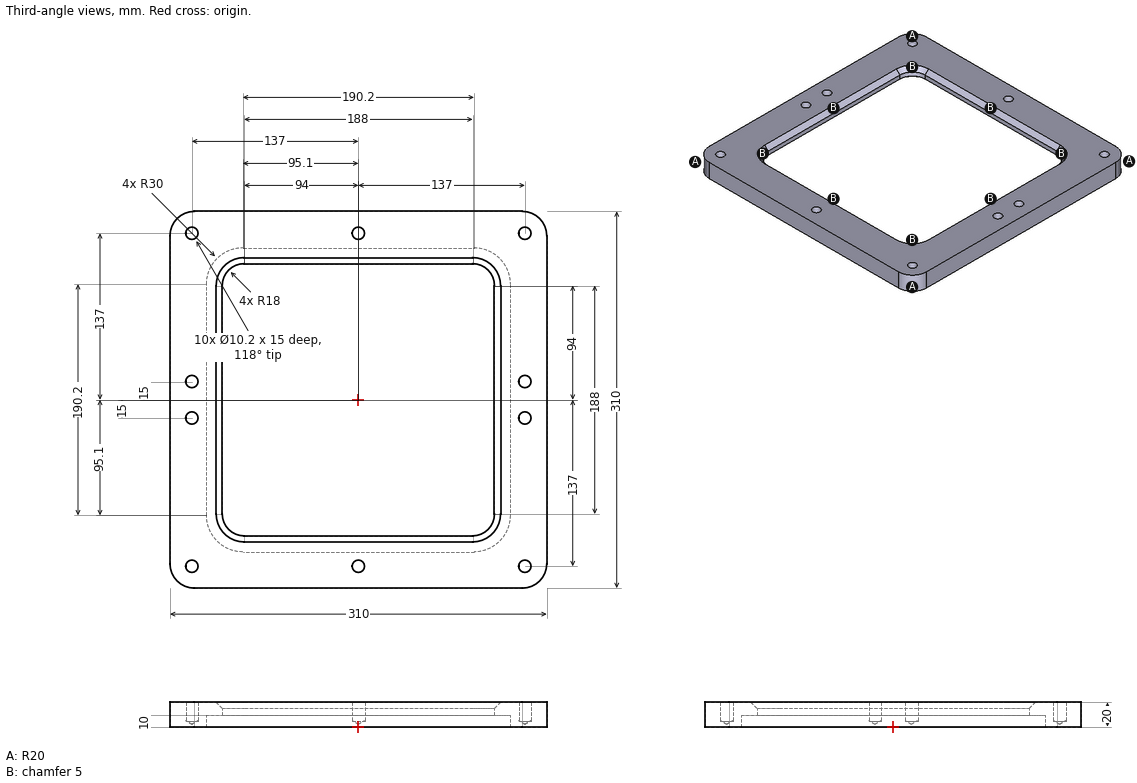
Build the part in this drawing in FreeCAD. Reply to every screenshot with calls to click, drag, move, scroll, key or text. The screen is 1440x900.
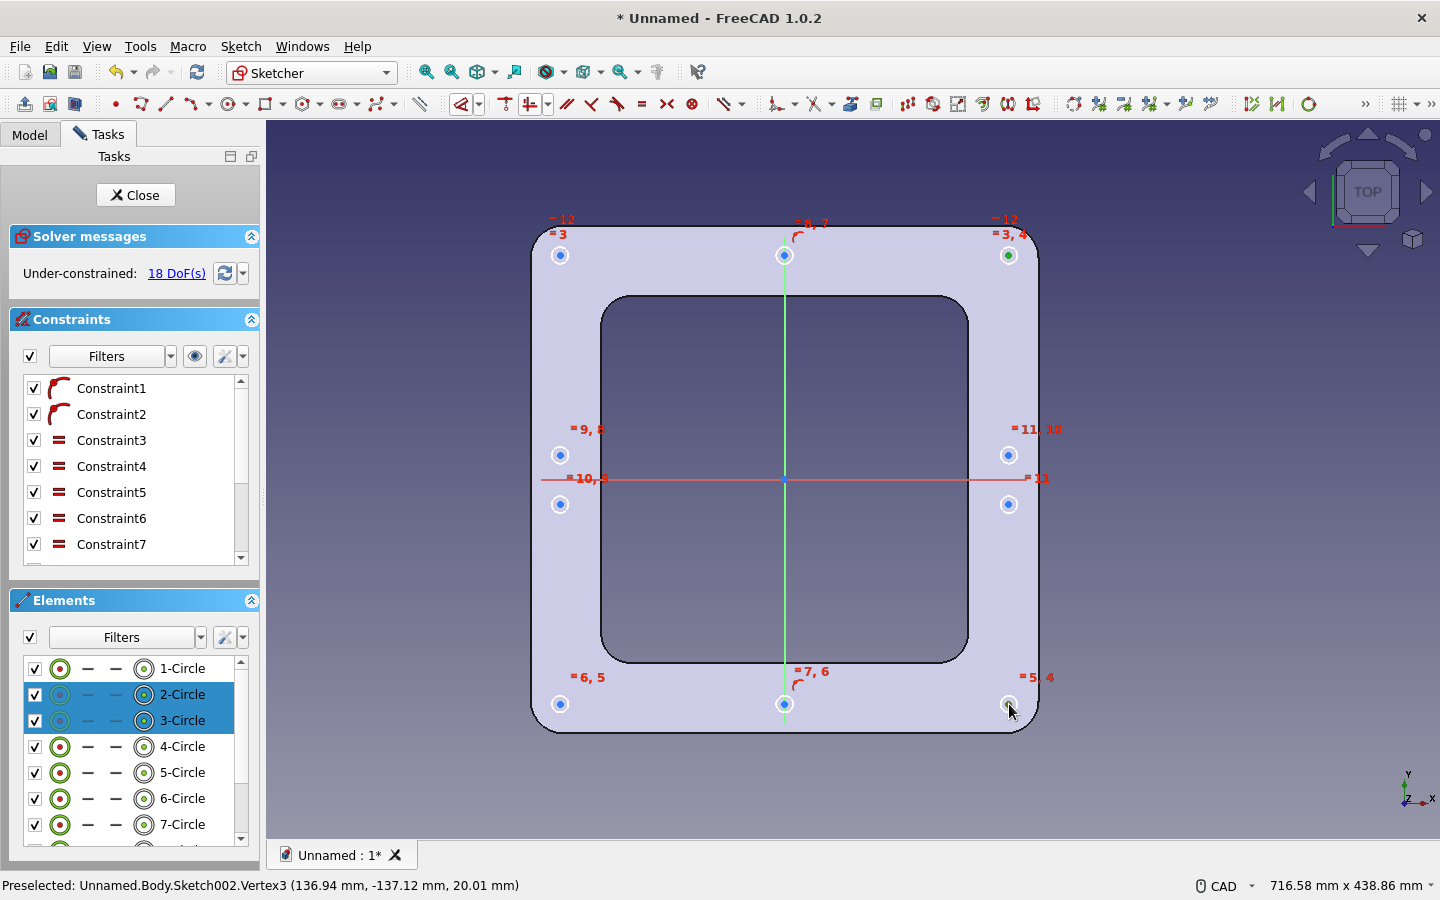
key(v)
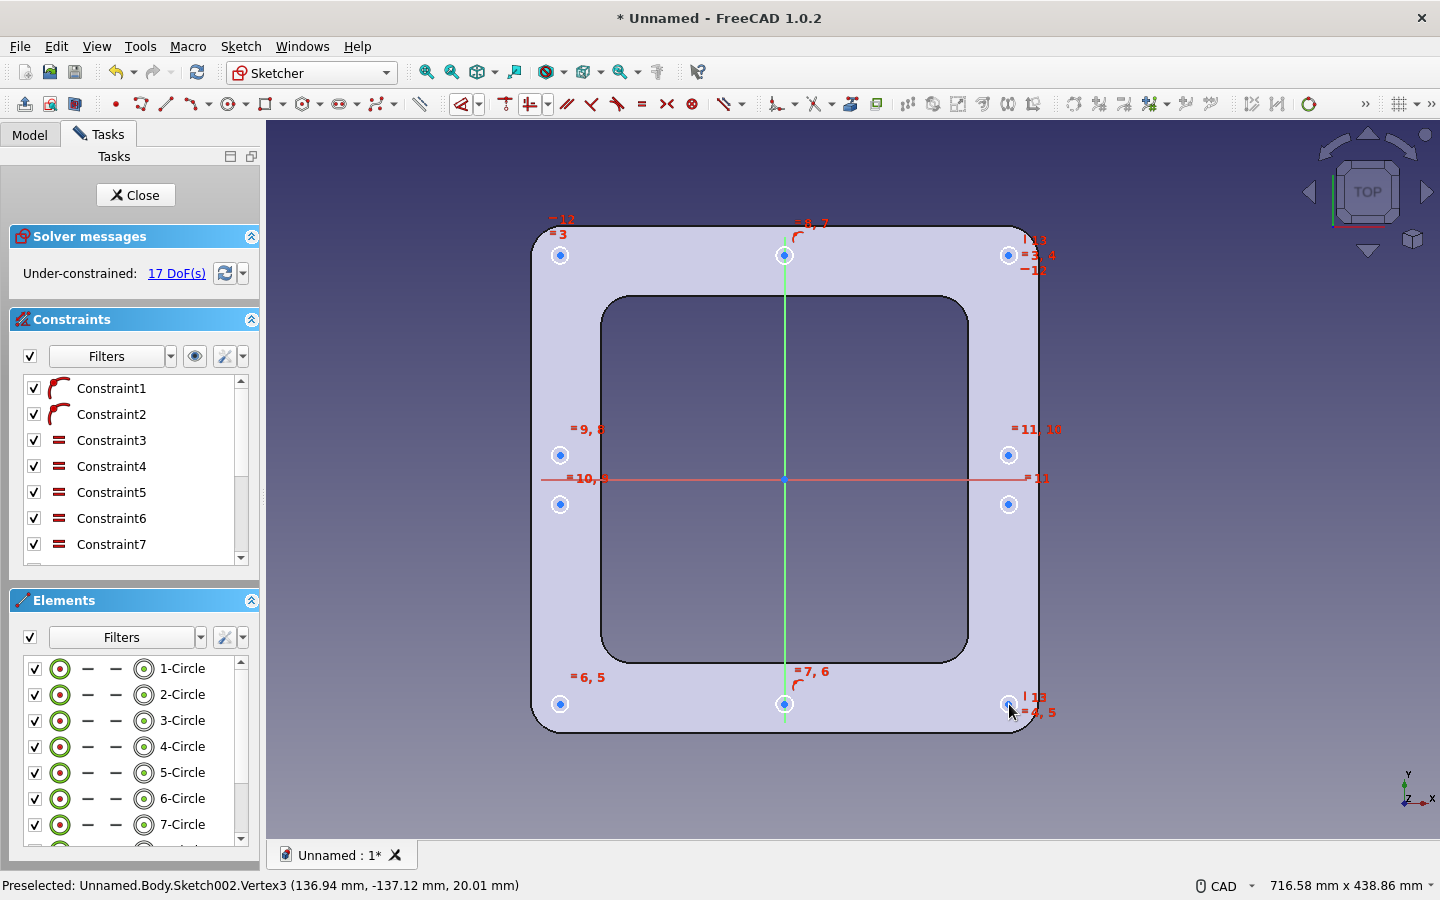
click(560, 255)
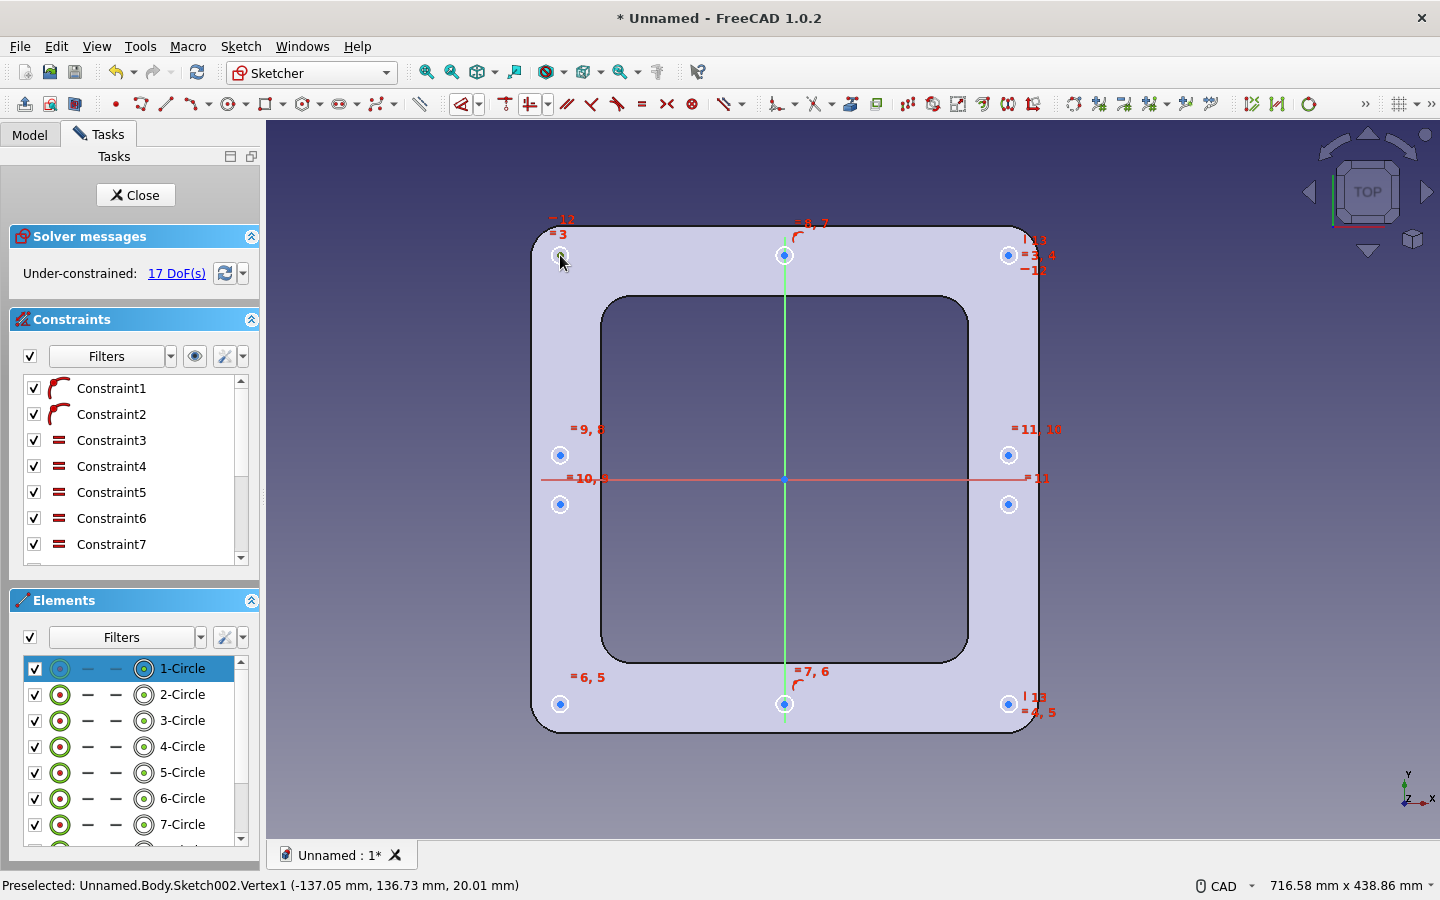
click(560, 704)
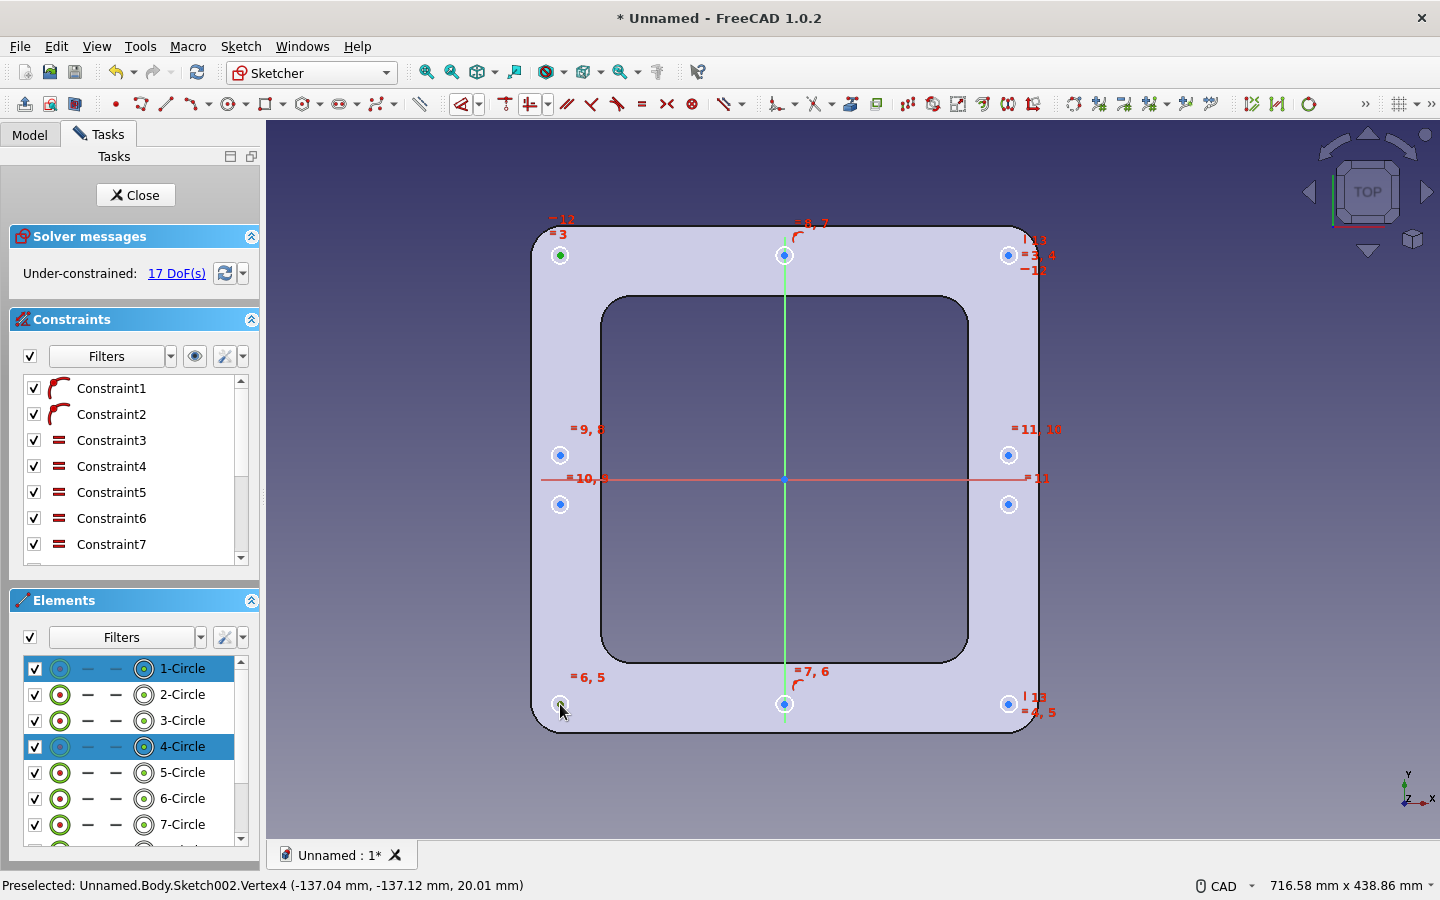
click(548, 104)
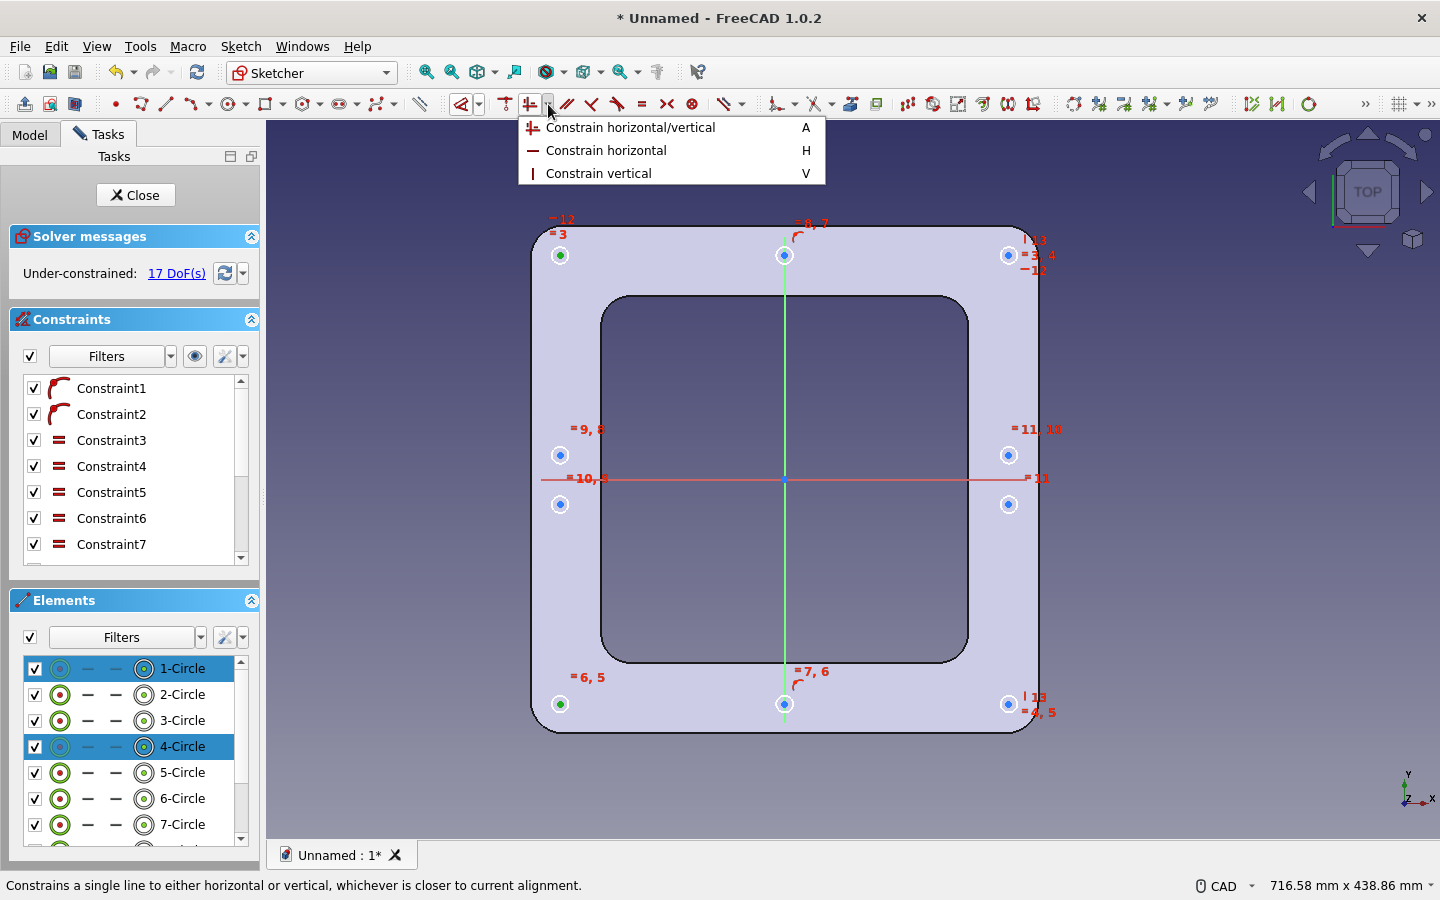
click(672, 174)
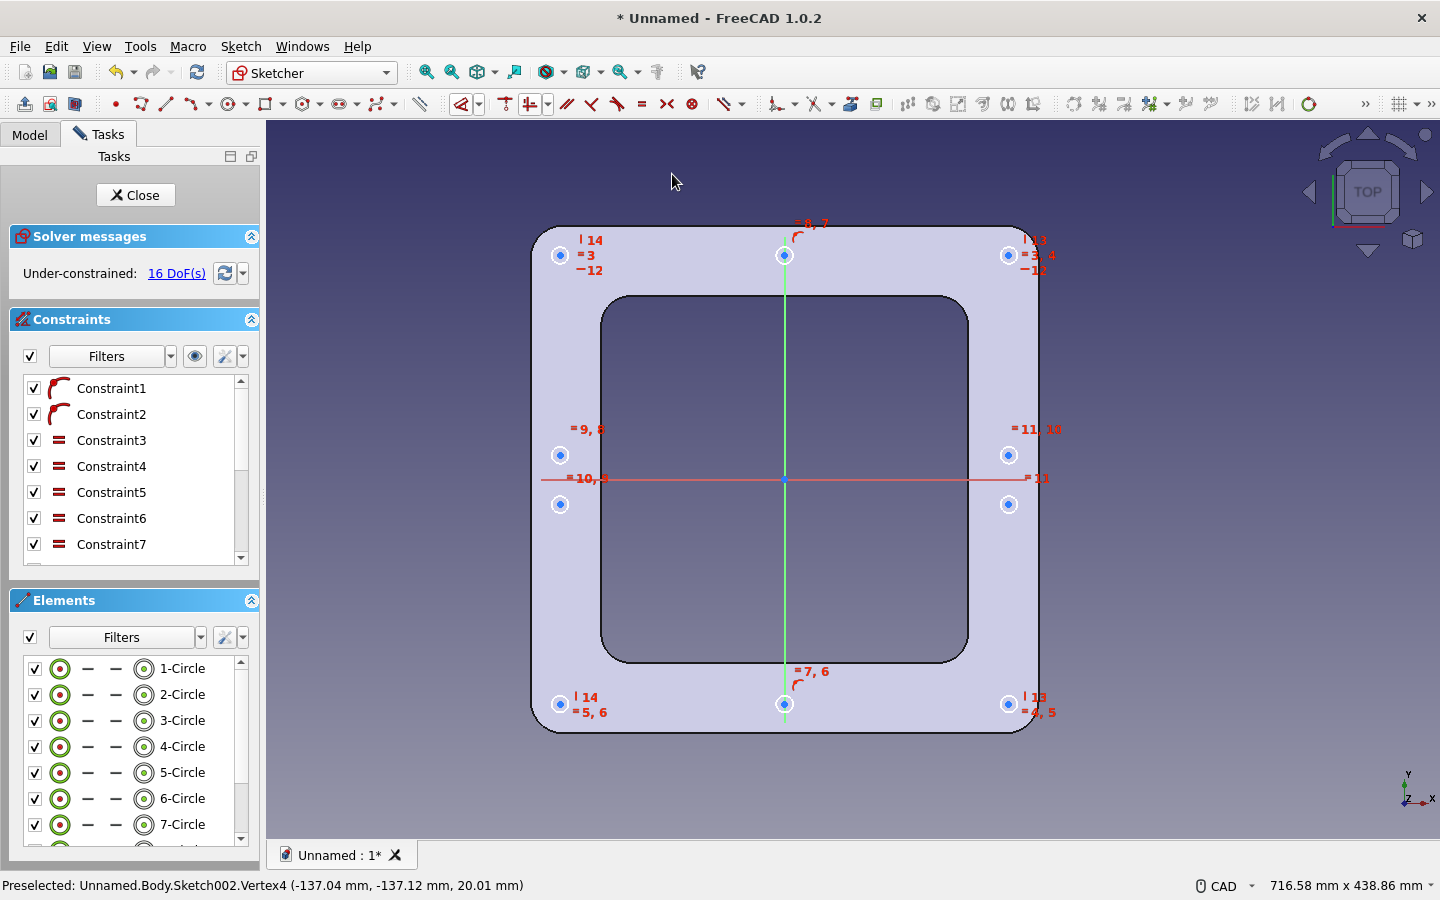
click(1009, 704)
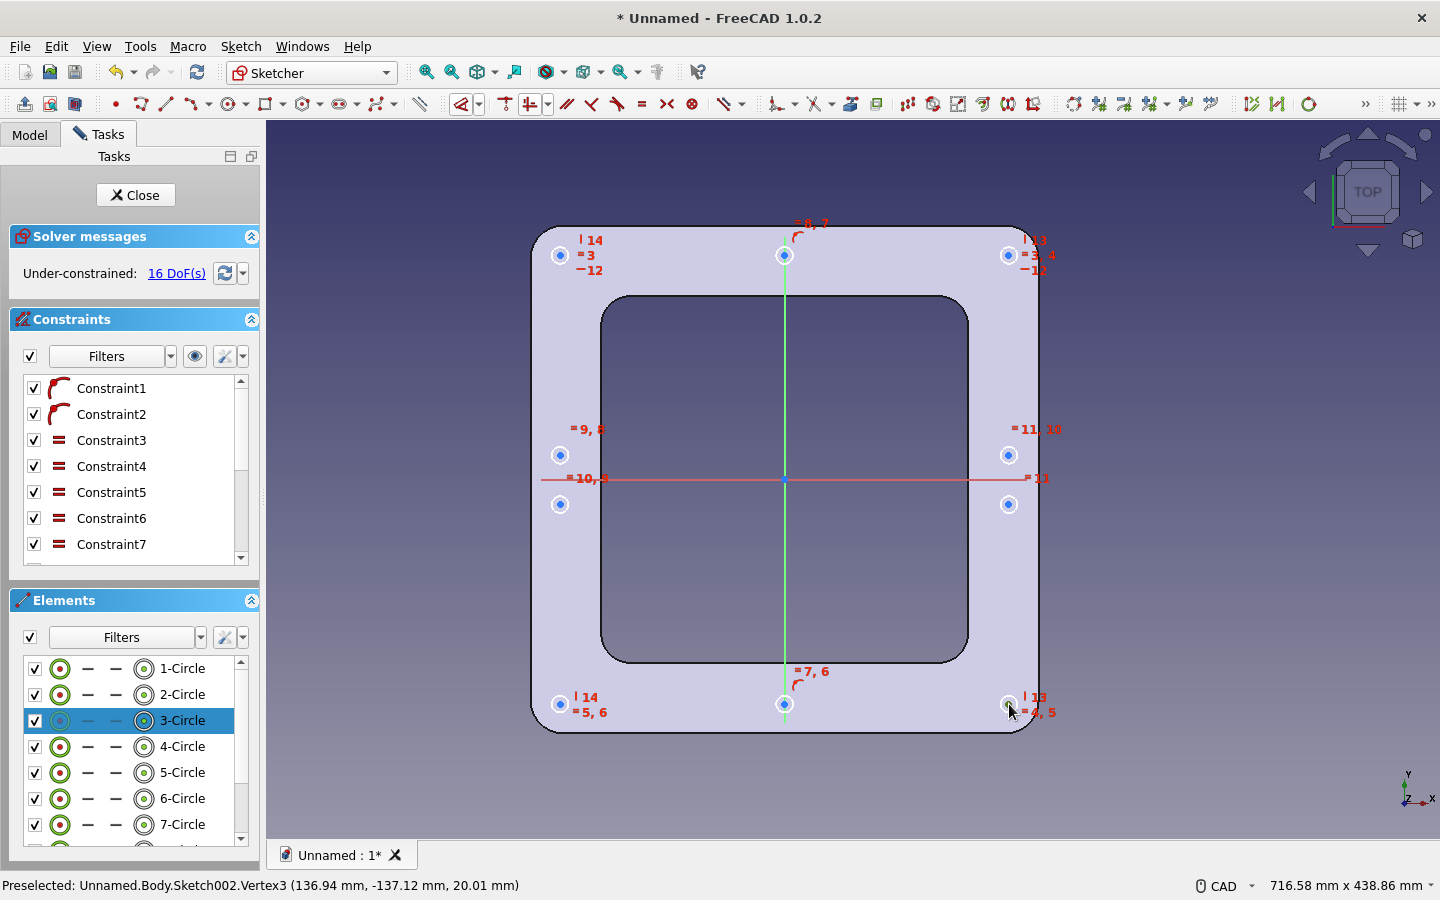
click(560, 704)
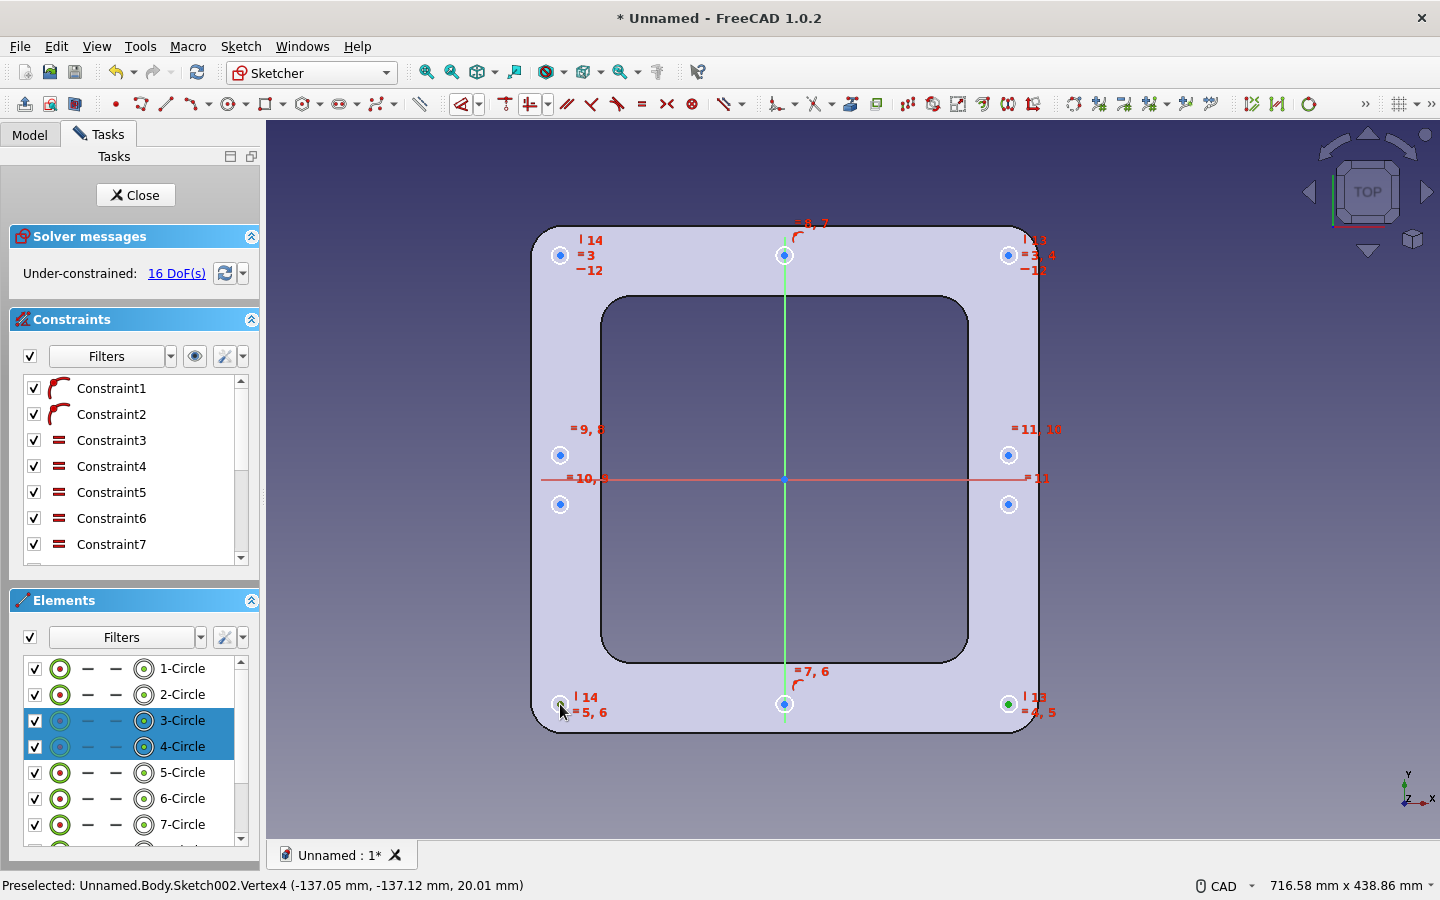
click(548, 104)